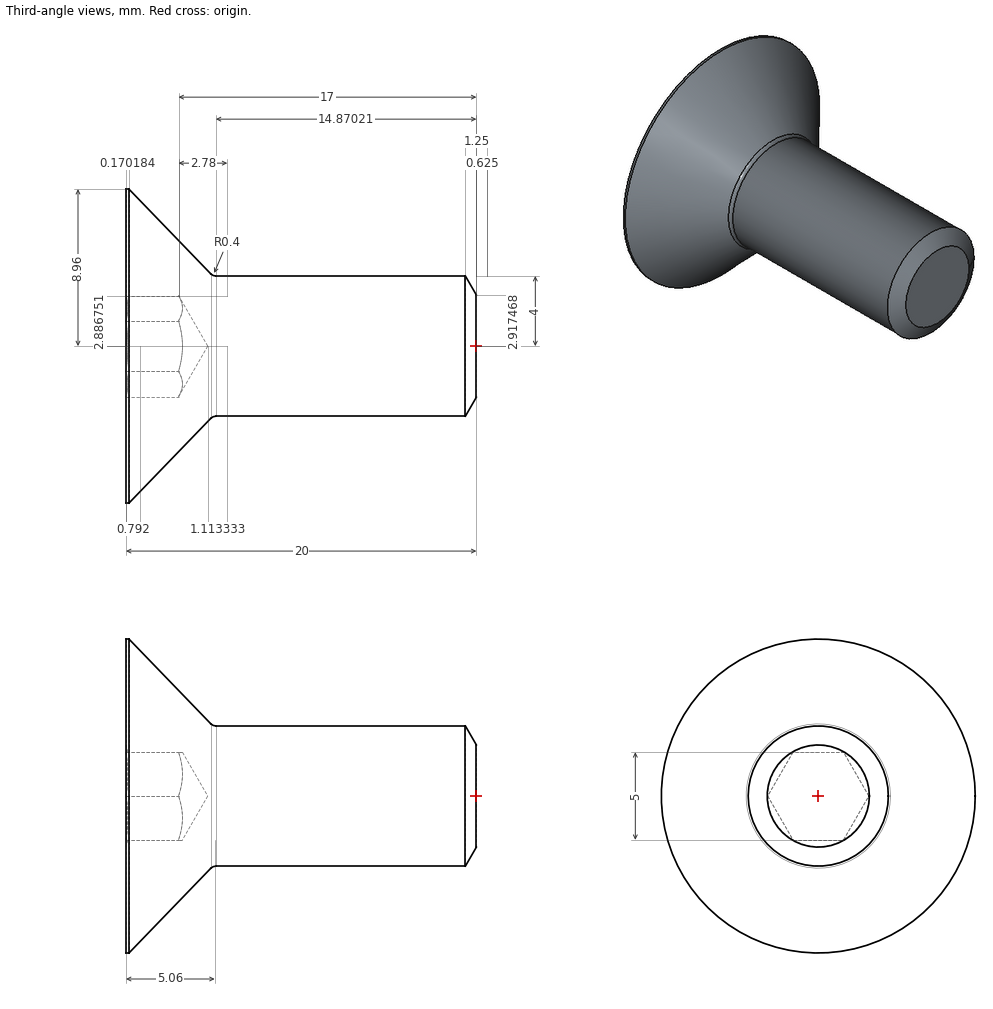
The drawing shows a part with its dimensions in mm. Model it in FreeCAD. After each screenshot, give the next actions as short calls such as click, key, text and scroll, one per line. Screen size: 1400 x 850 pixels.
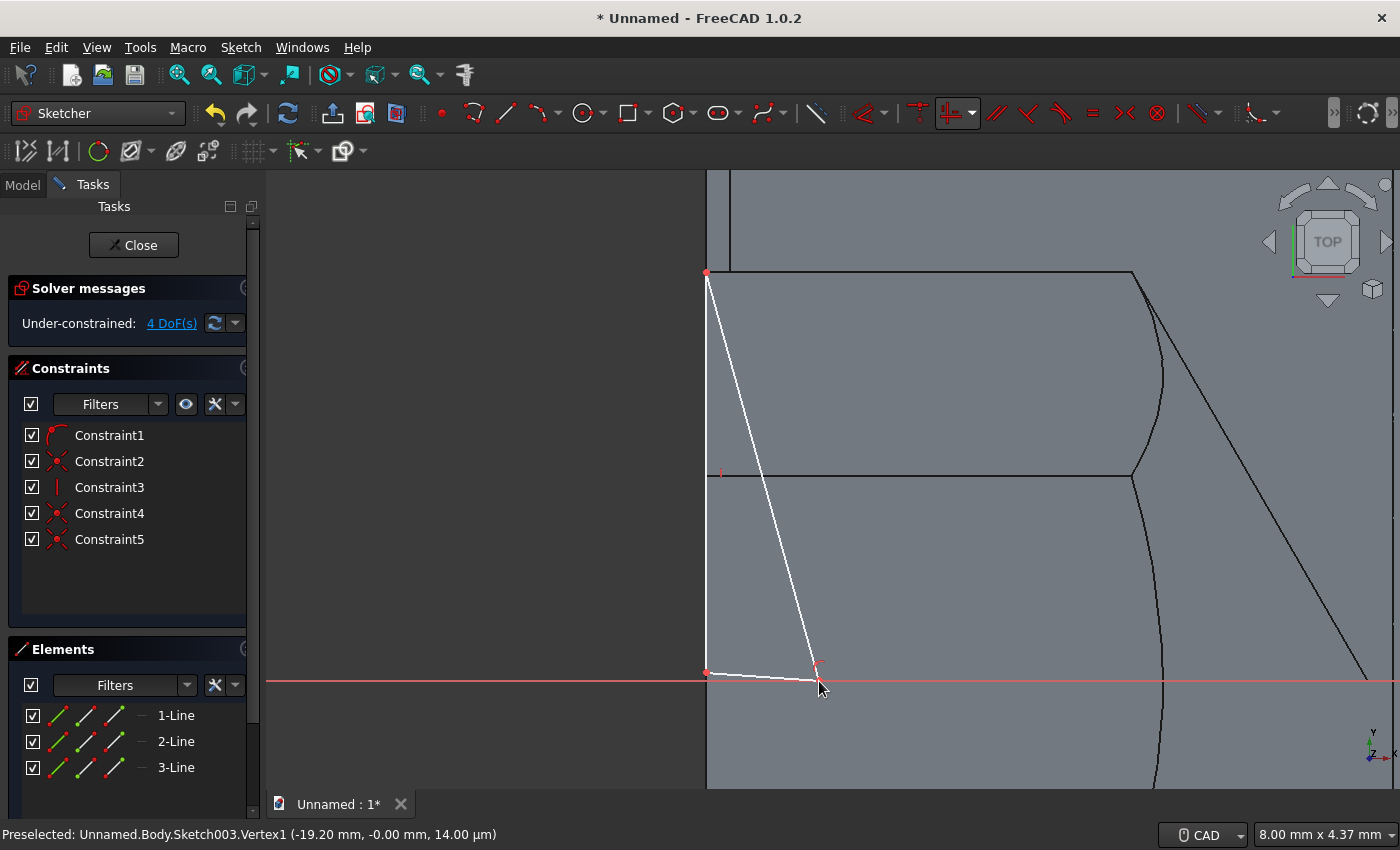
click(785, 679)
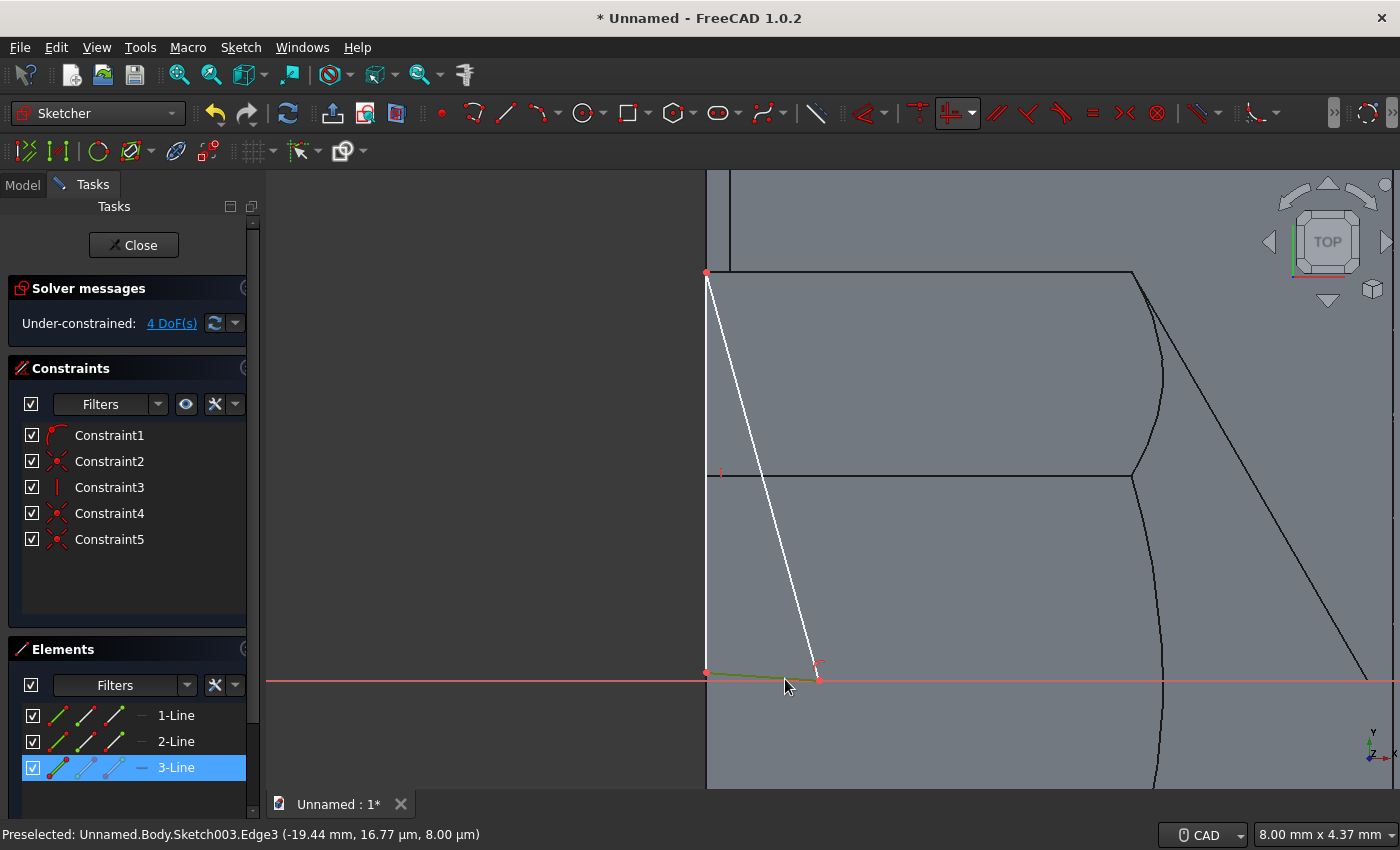
click(974, 114)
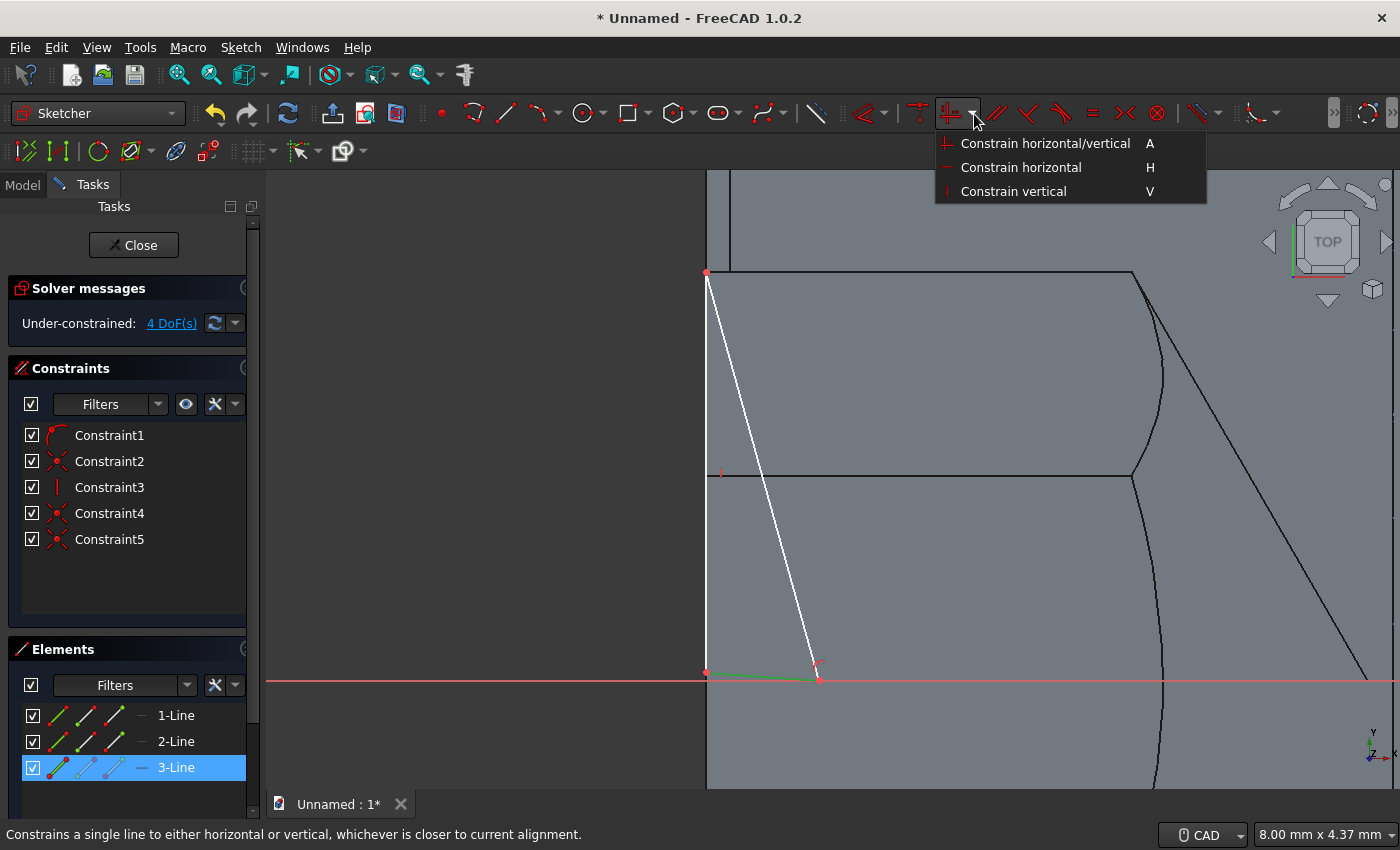
click(1071, 167)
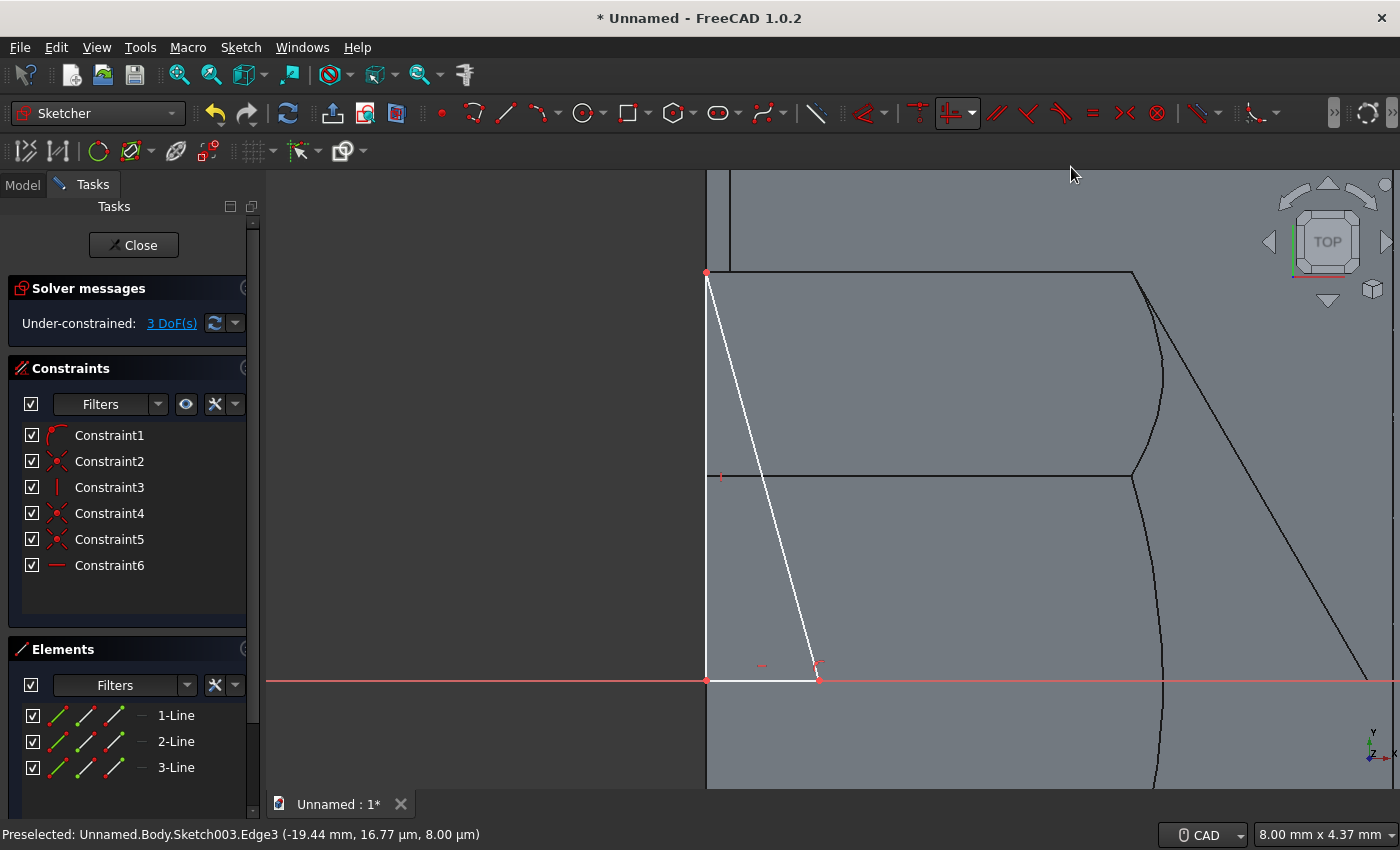
click(864, 114)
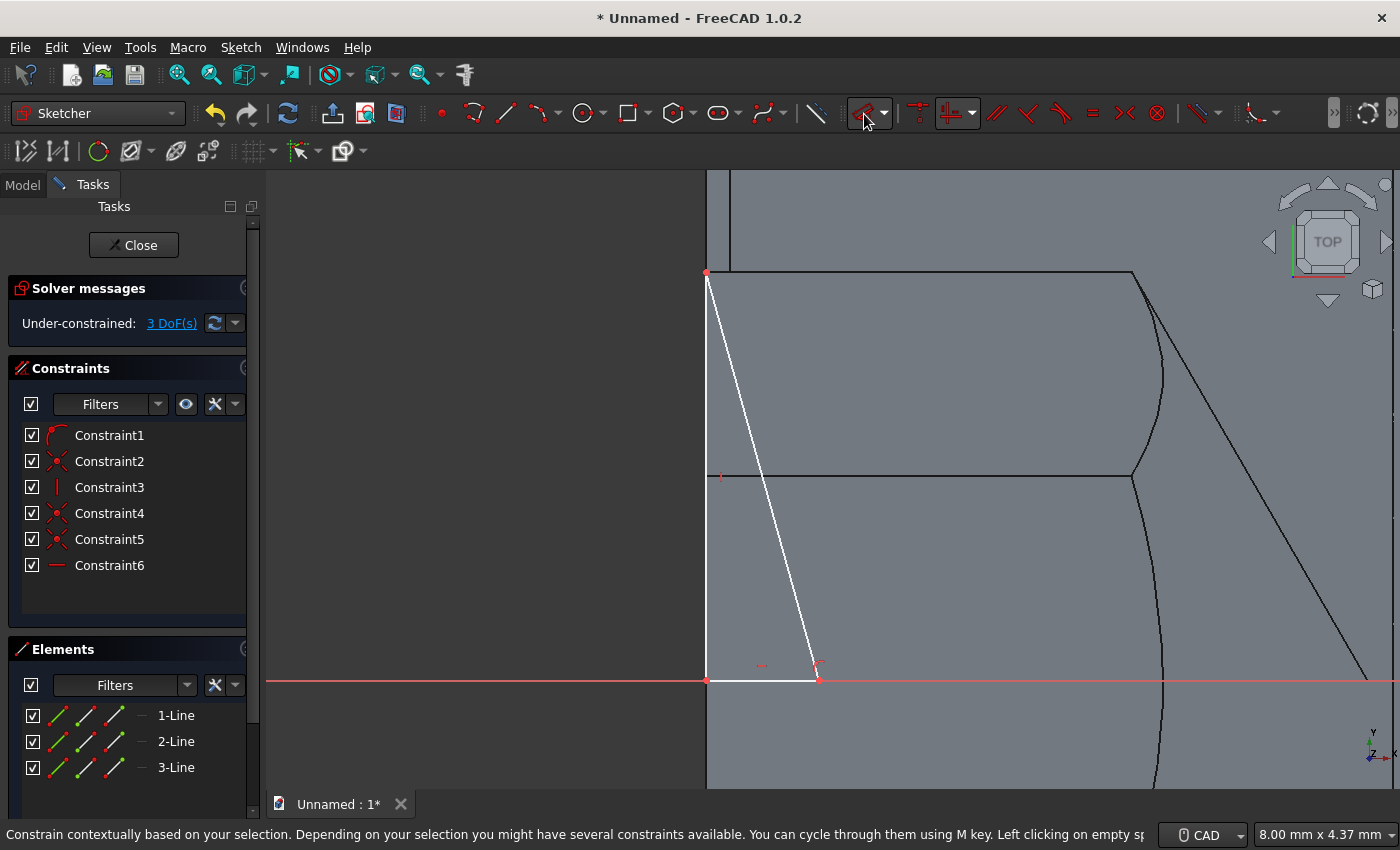
click(706, 273)
click(971, 715)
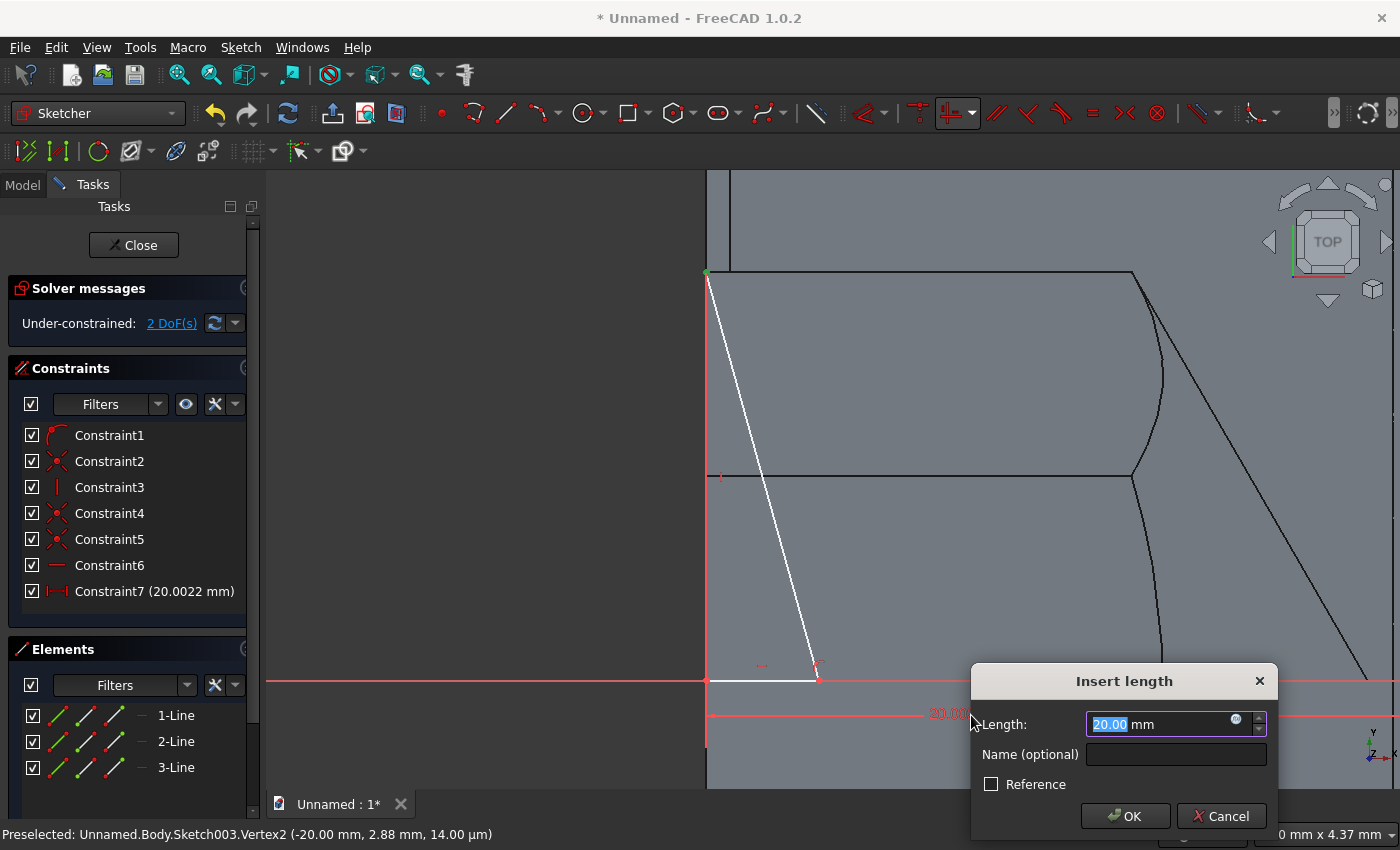
text(20)
key(Return)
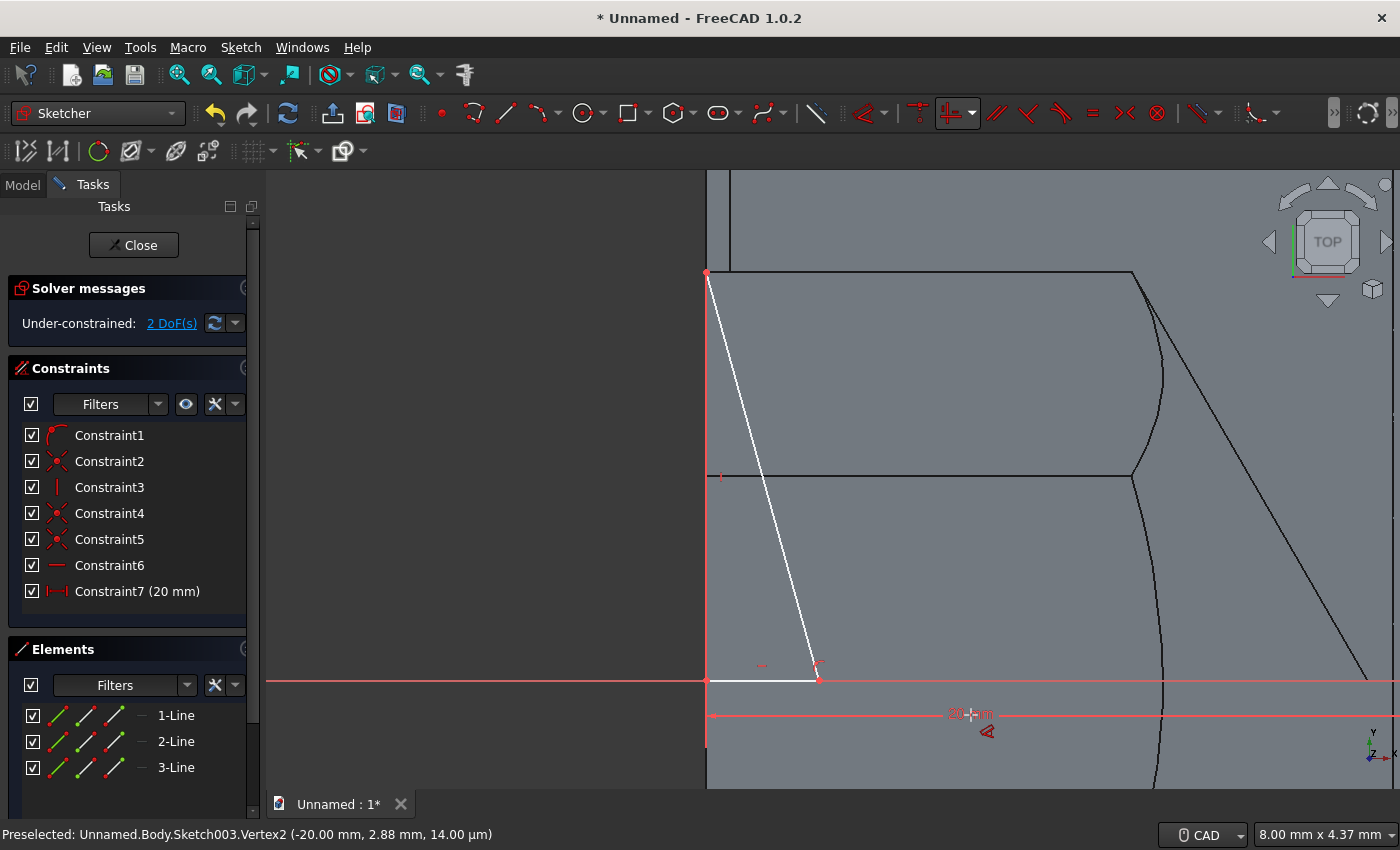
click(740, 681)
click(763, 715)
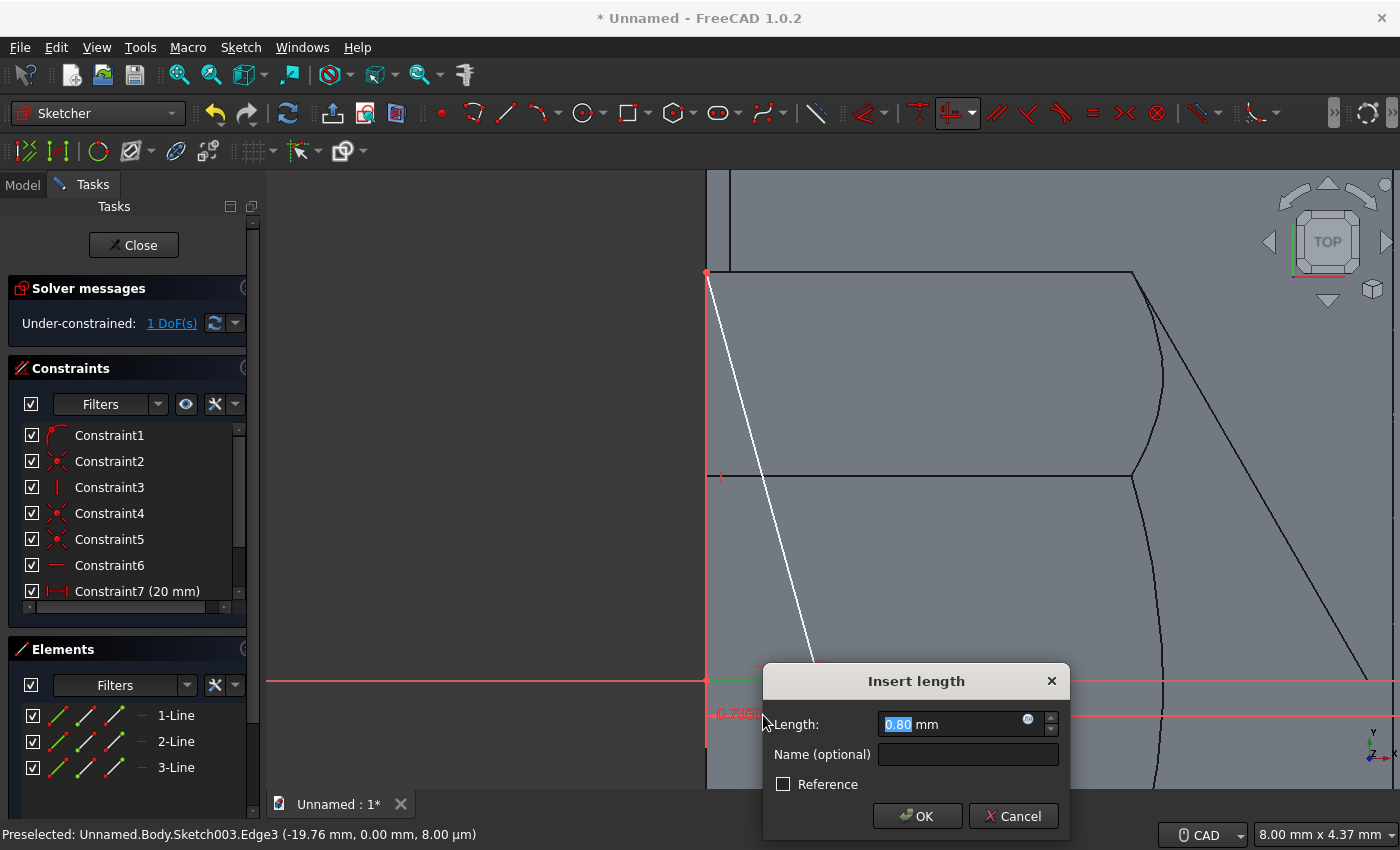
text(0.792)
key(Return)